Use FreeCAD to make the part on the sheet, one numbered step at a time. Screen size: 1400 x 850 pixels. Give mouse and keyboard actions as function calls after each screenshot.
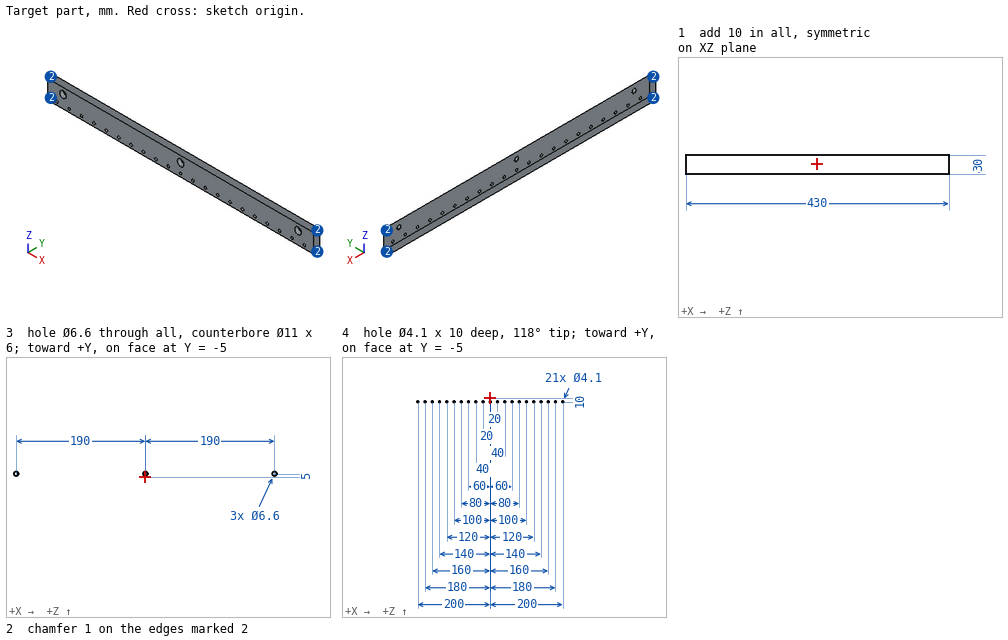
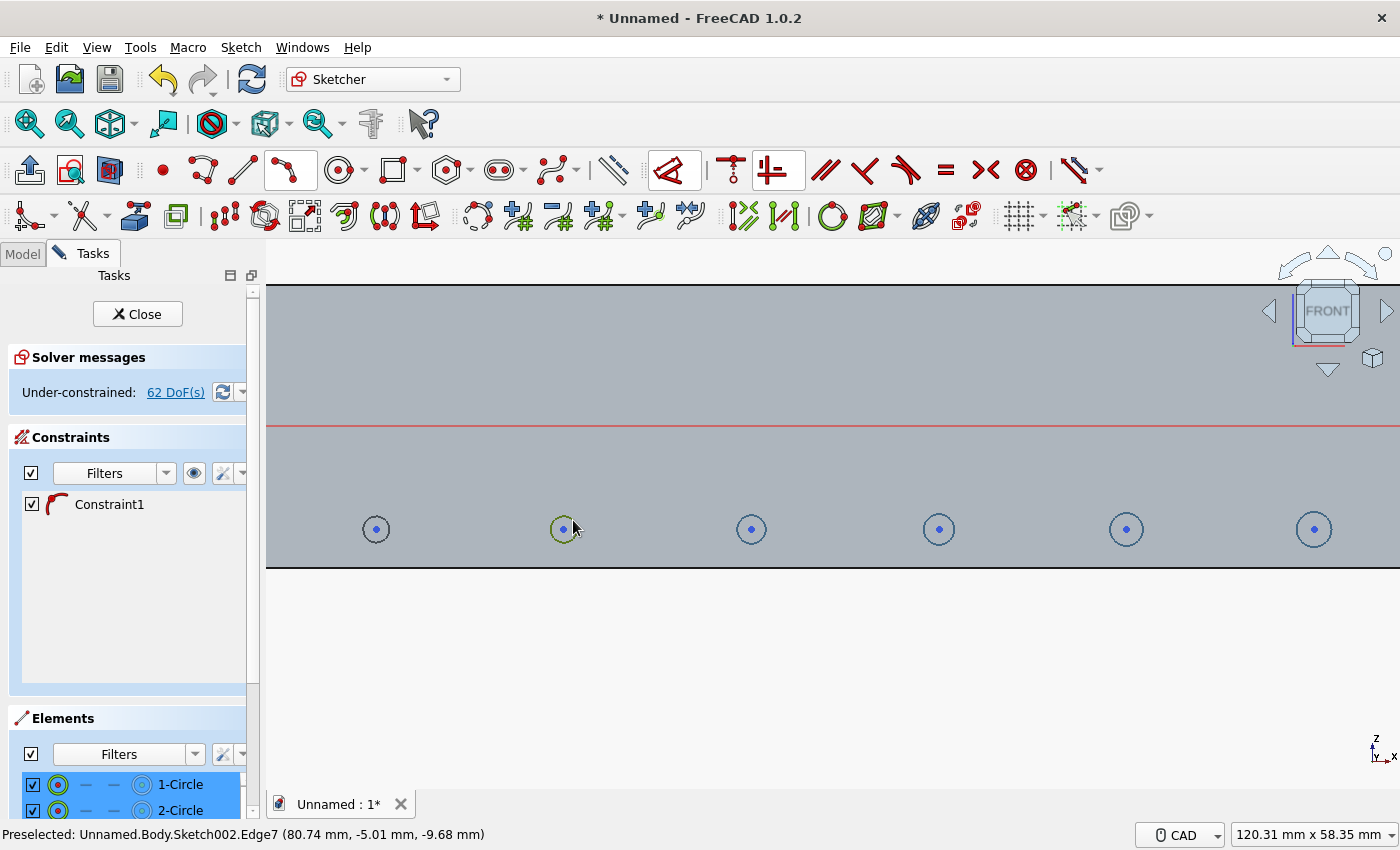
click(386, 520)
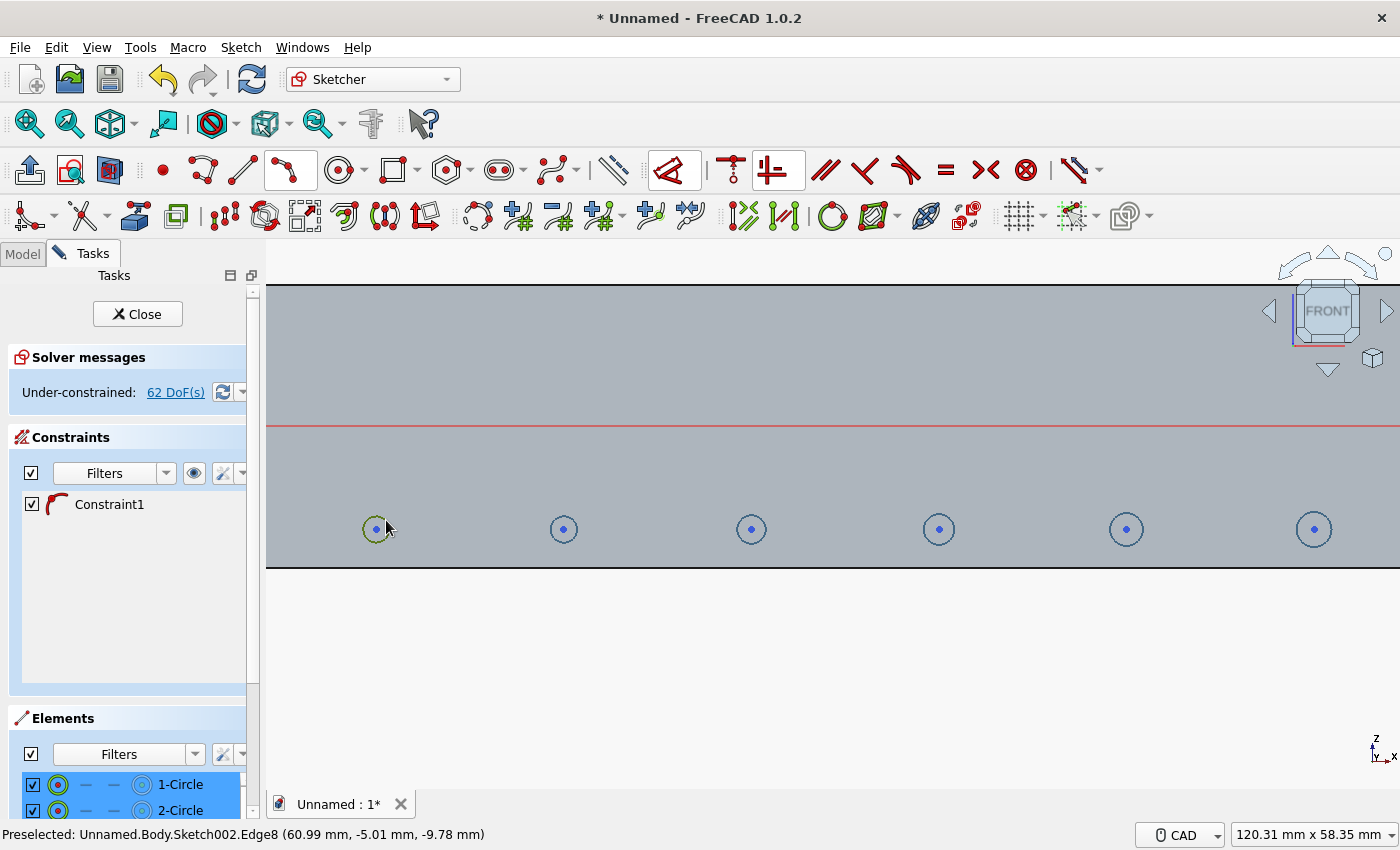
scroll(954, 520, down, 9)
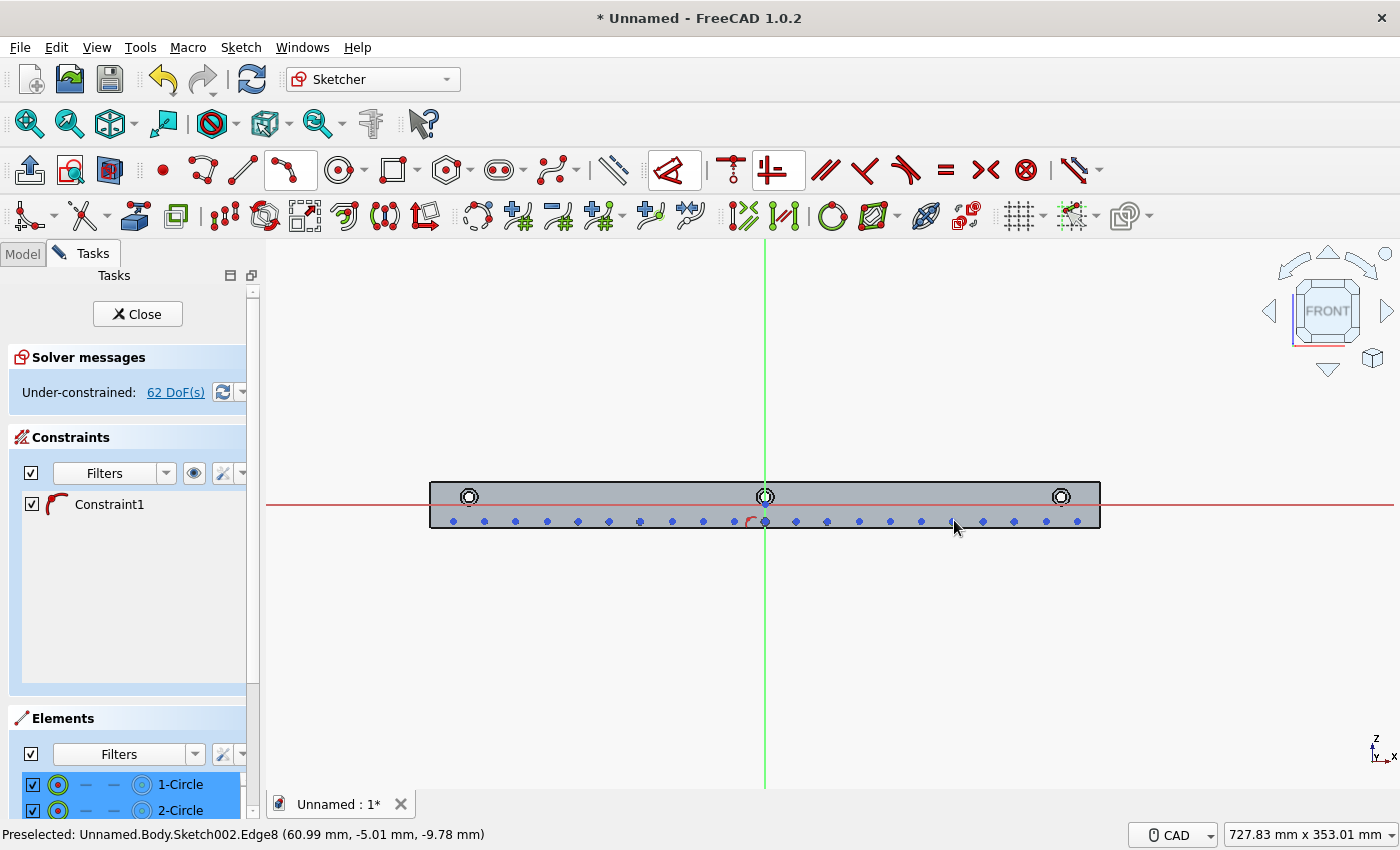
scroll(829, 520, up, 8)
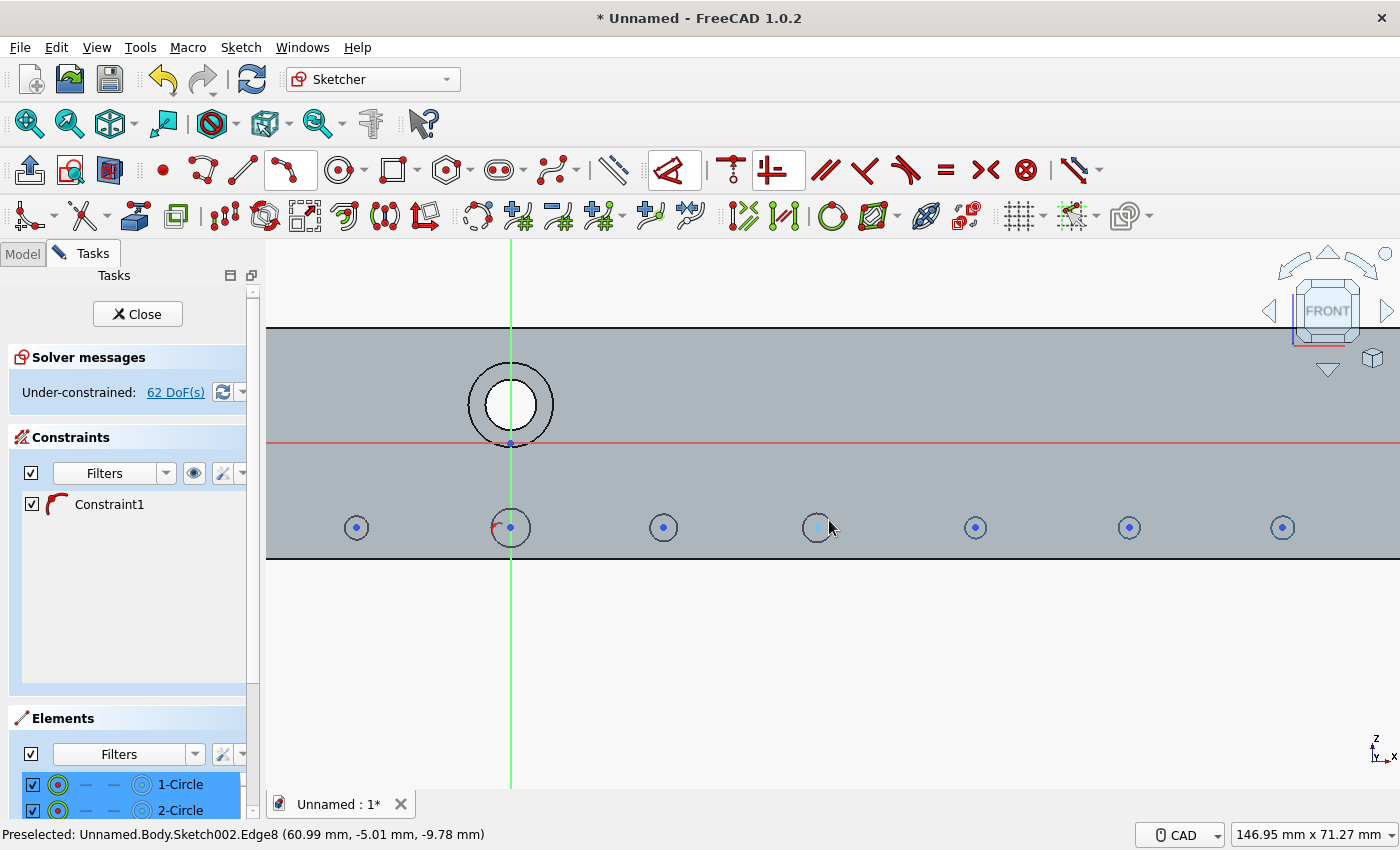
click(827, 518)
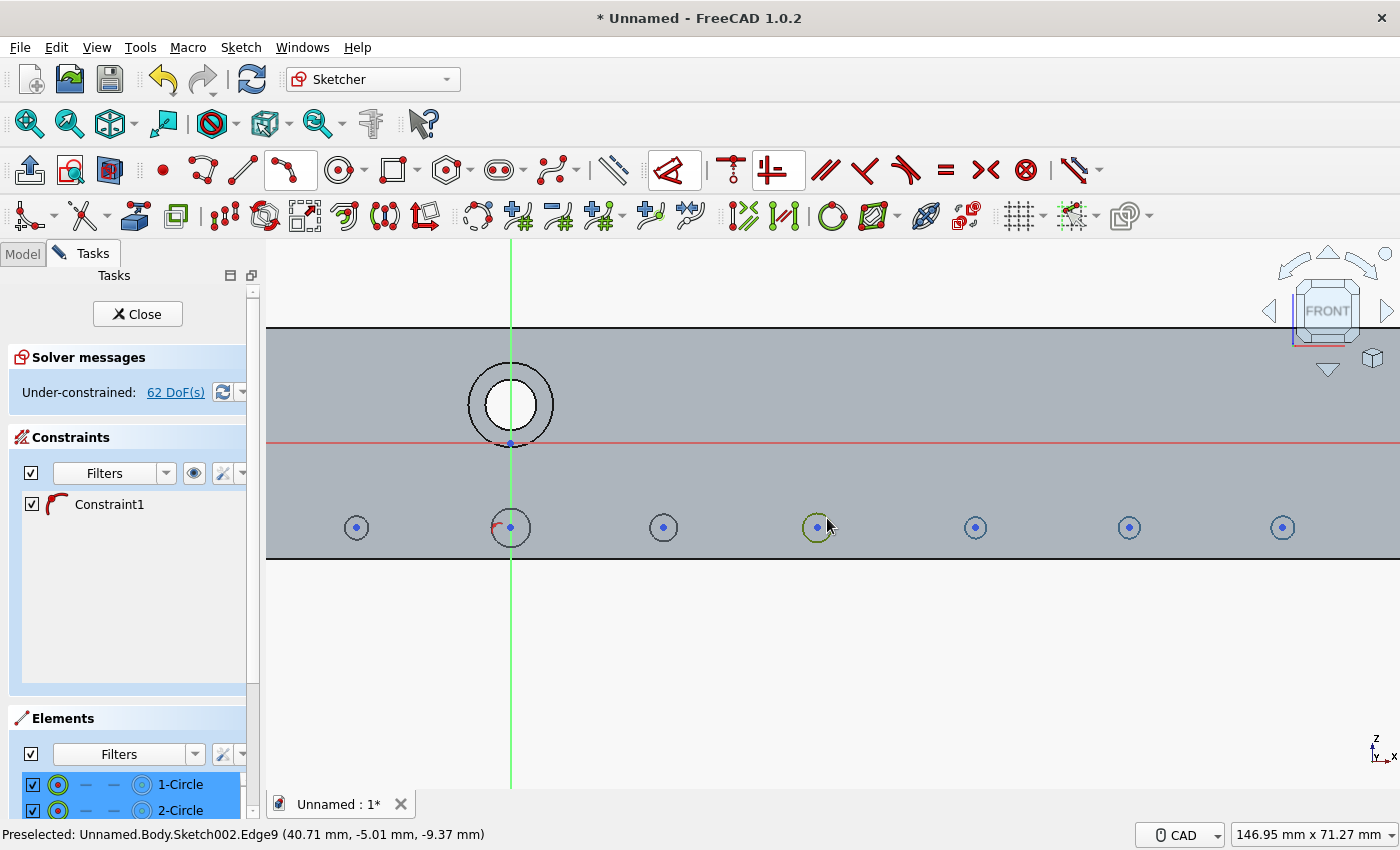
click(673, 518)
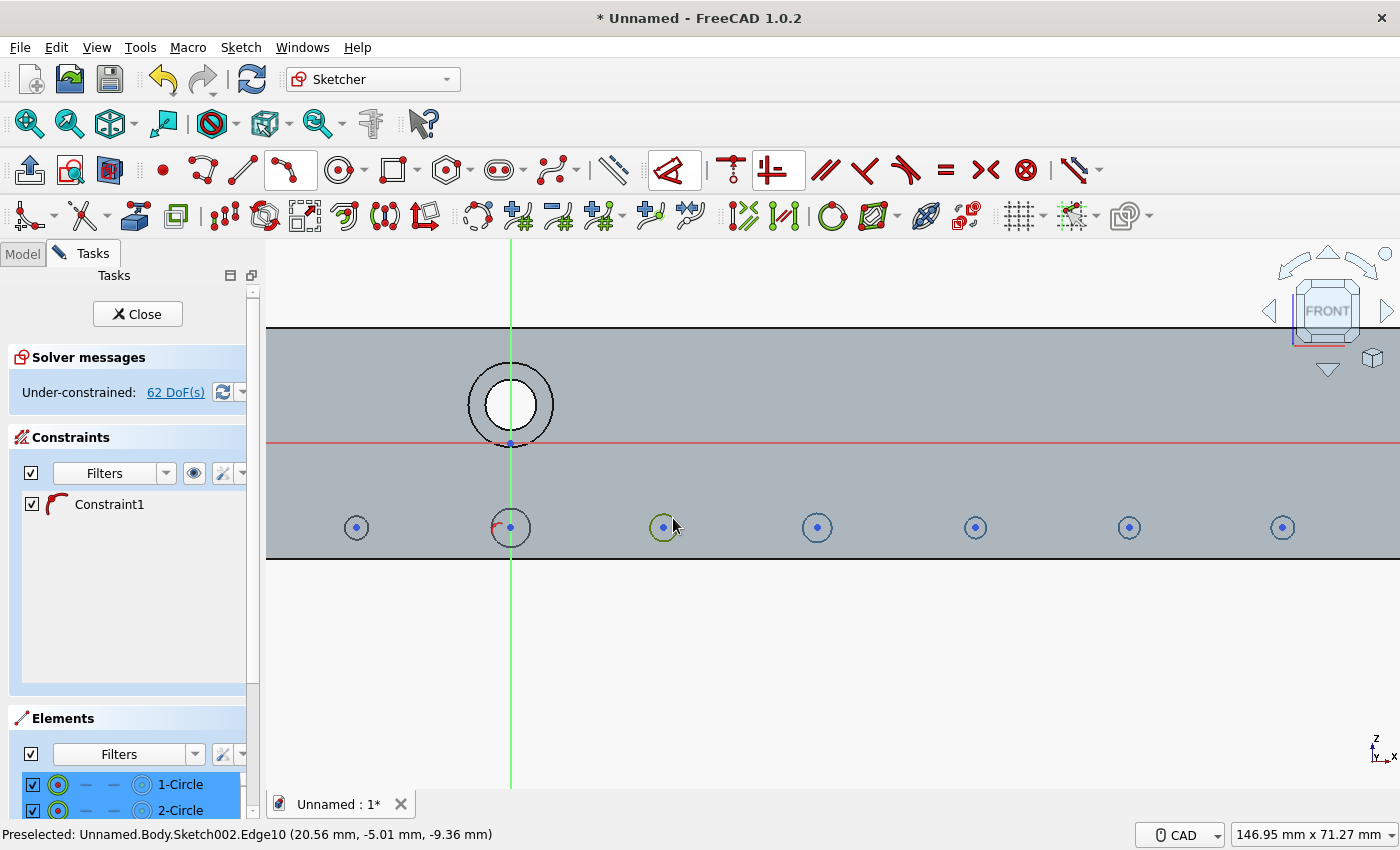
click(524, 514)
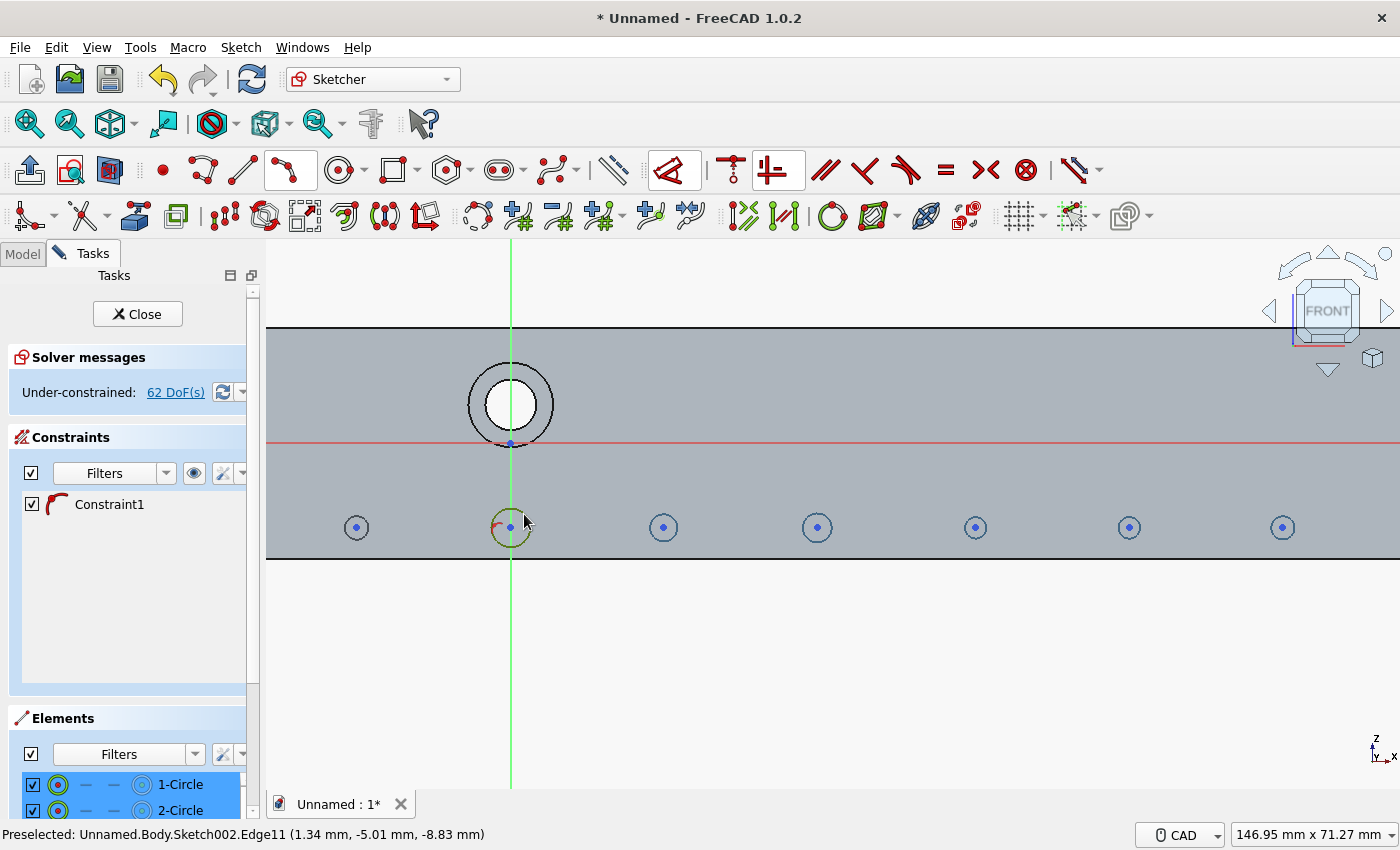
click(365, 520)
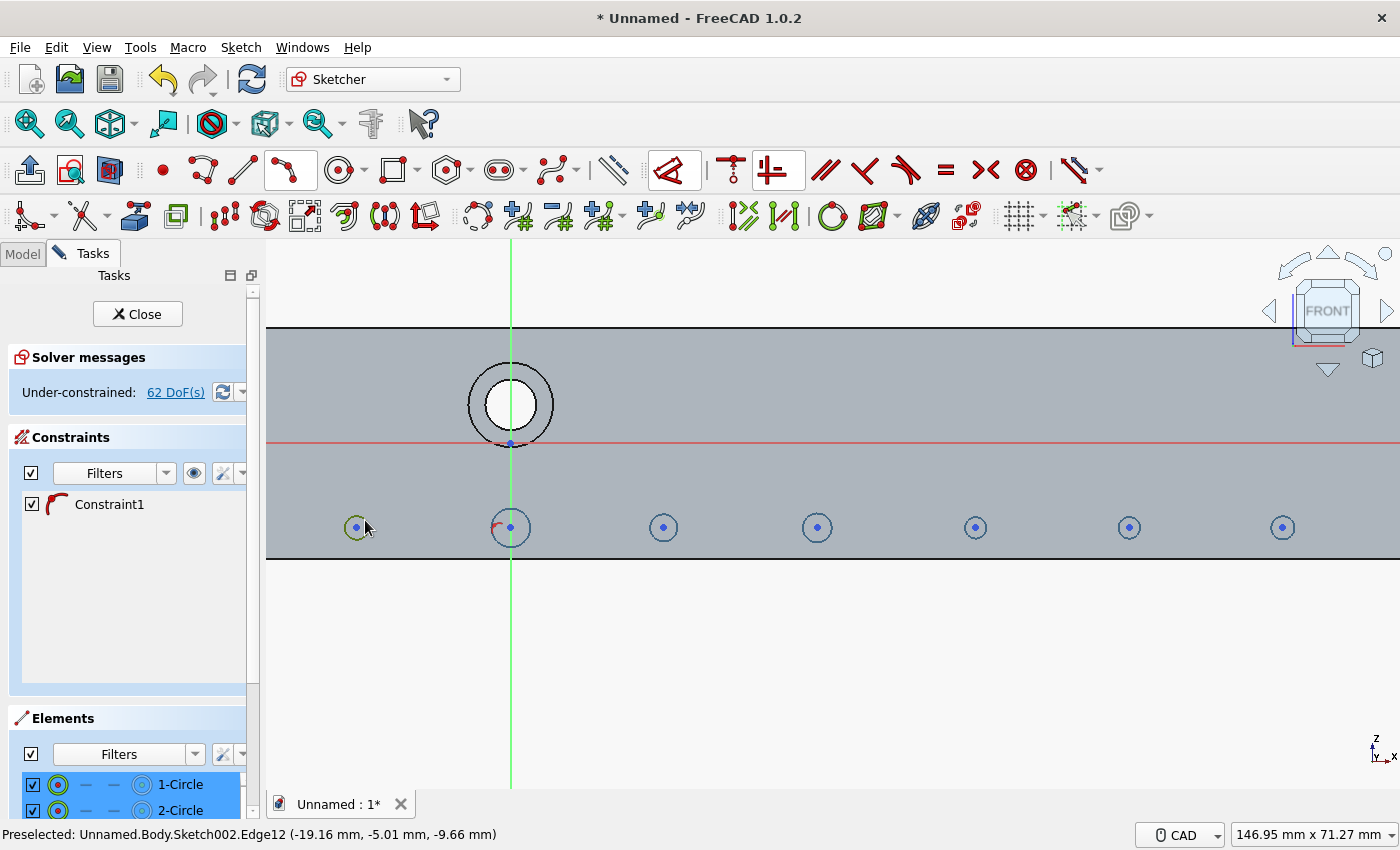
scroll(829, 520, down, 8)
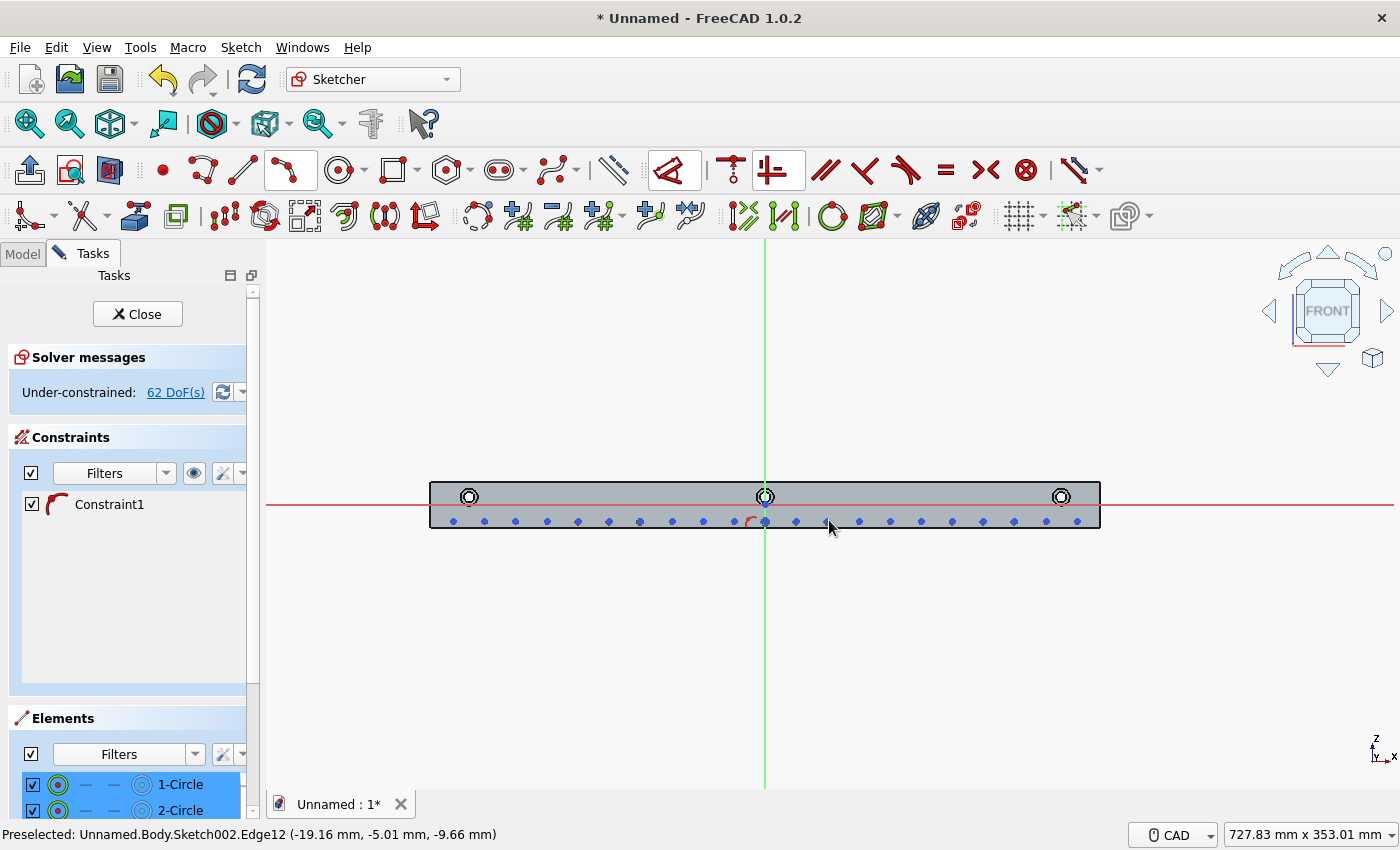
scroll(705, 520, up, 10)